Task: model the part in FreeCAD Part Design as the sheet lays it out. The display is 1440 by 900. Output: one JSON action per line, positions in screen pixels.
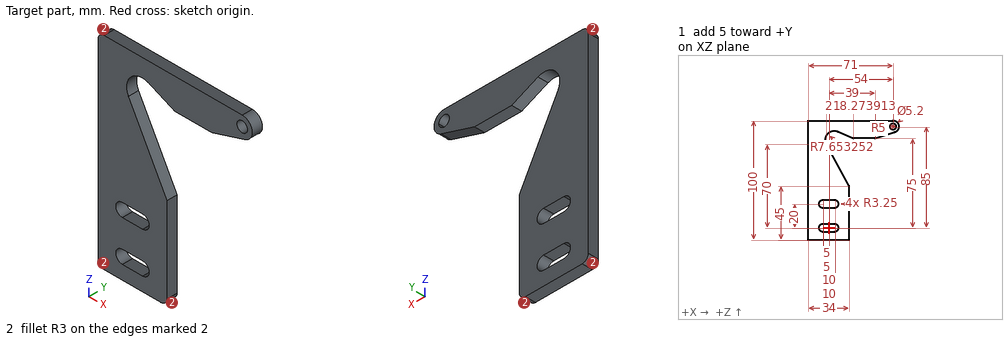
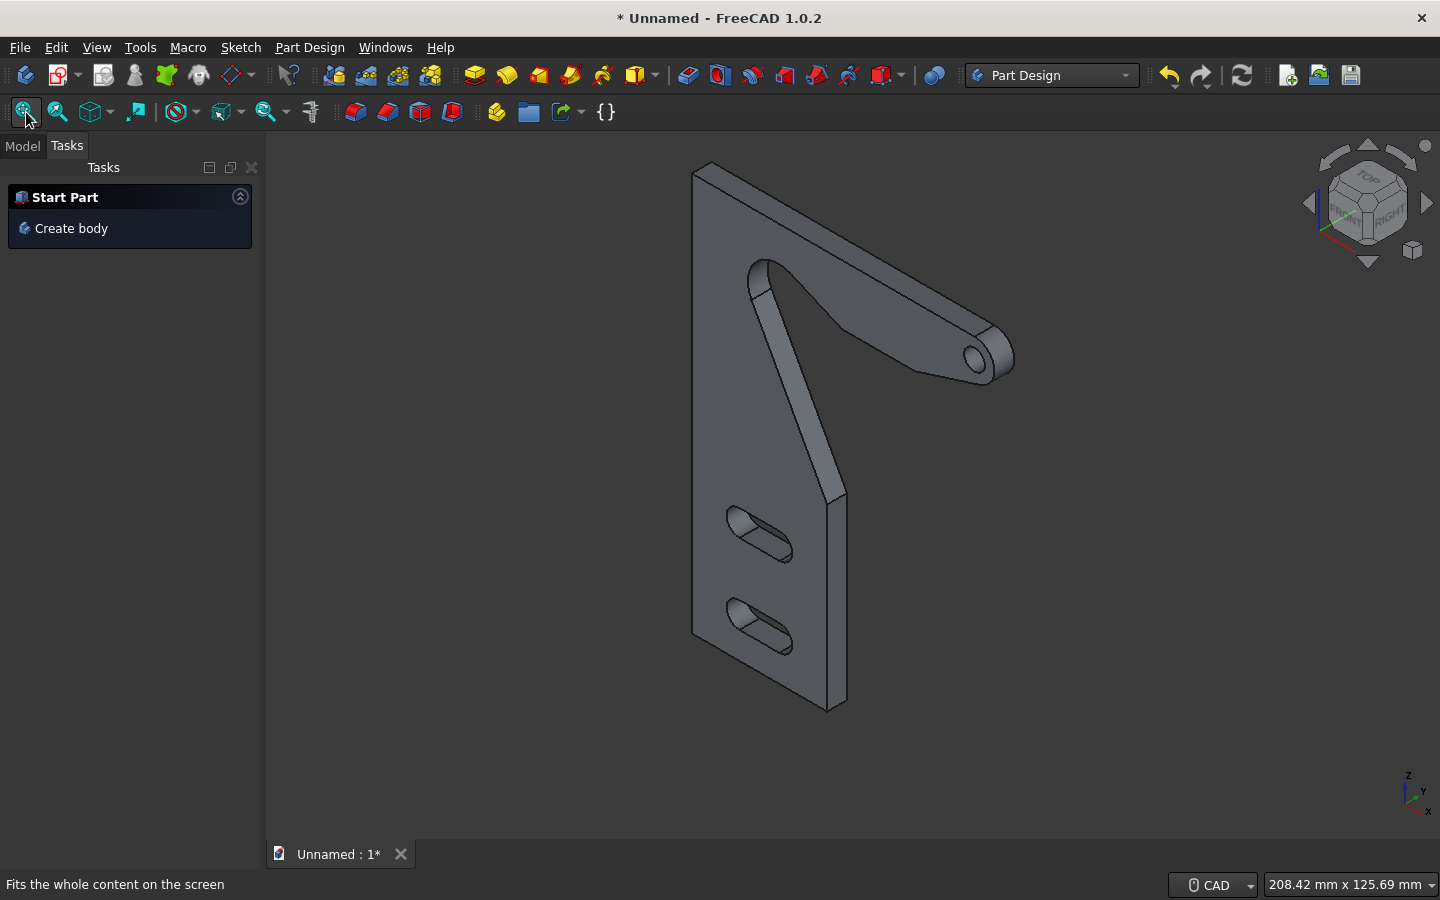
{"action": "key", "text": "2"}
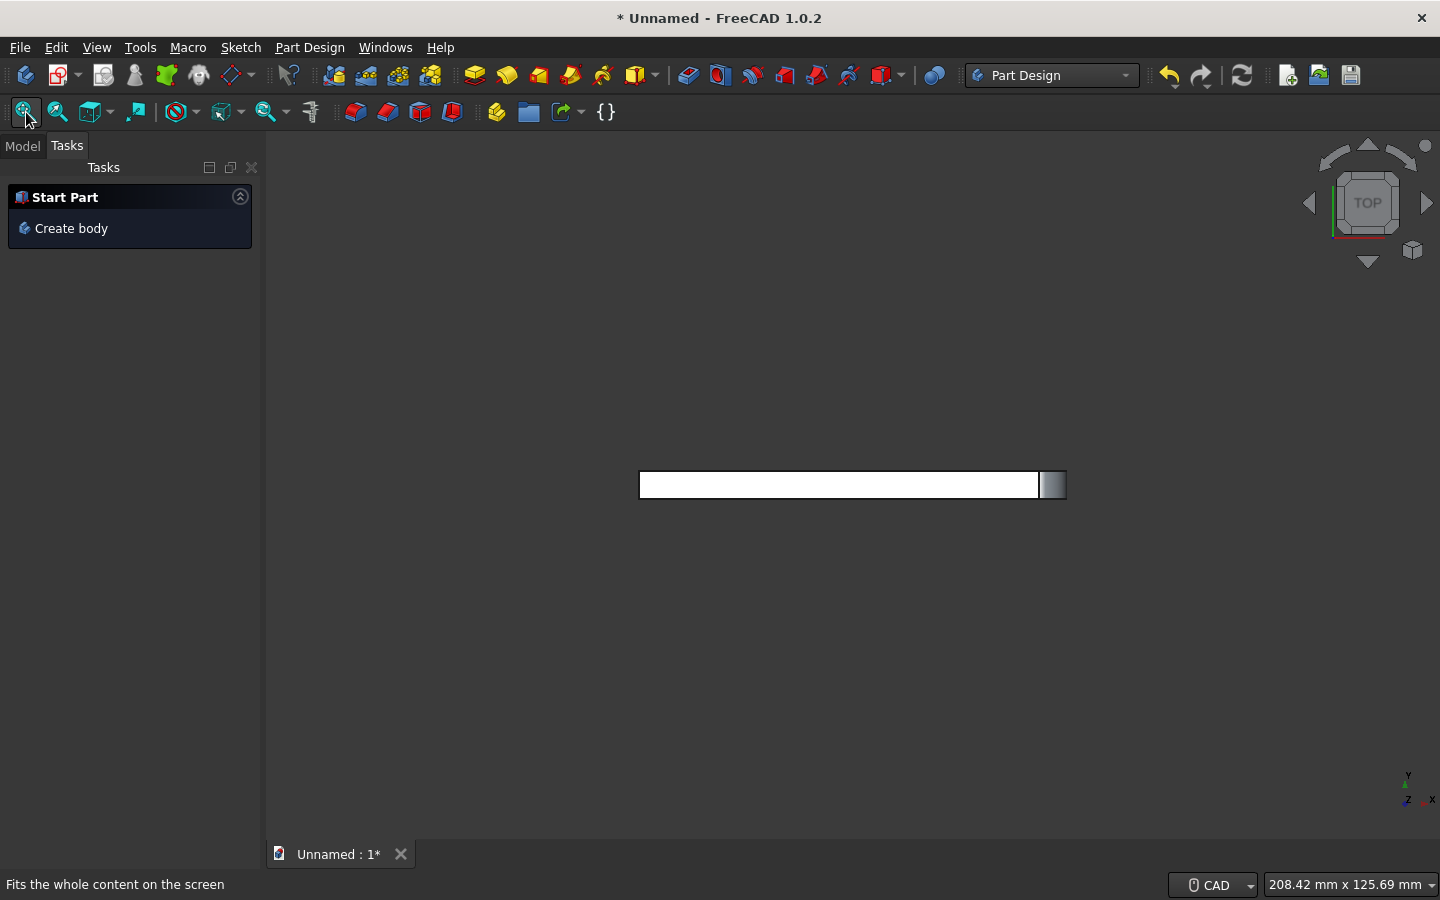
{"action": "left_click", "coordinate": [26, 112]}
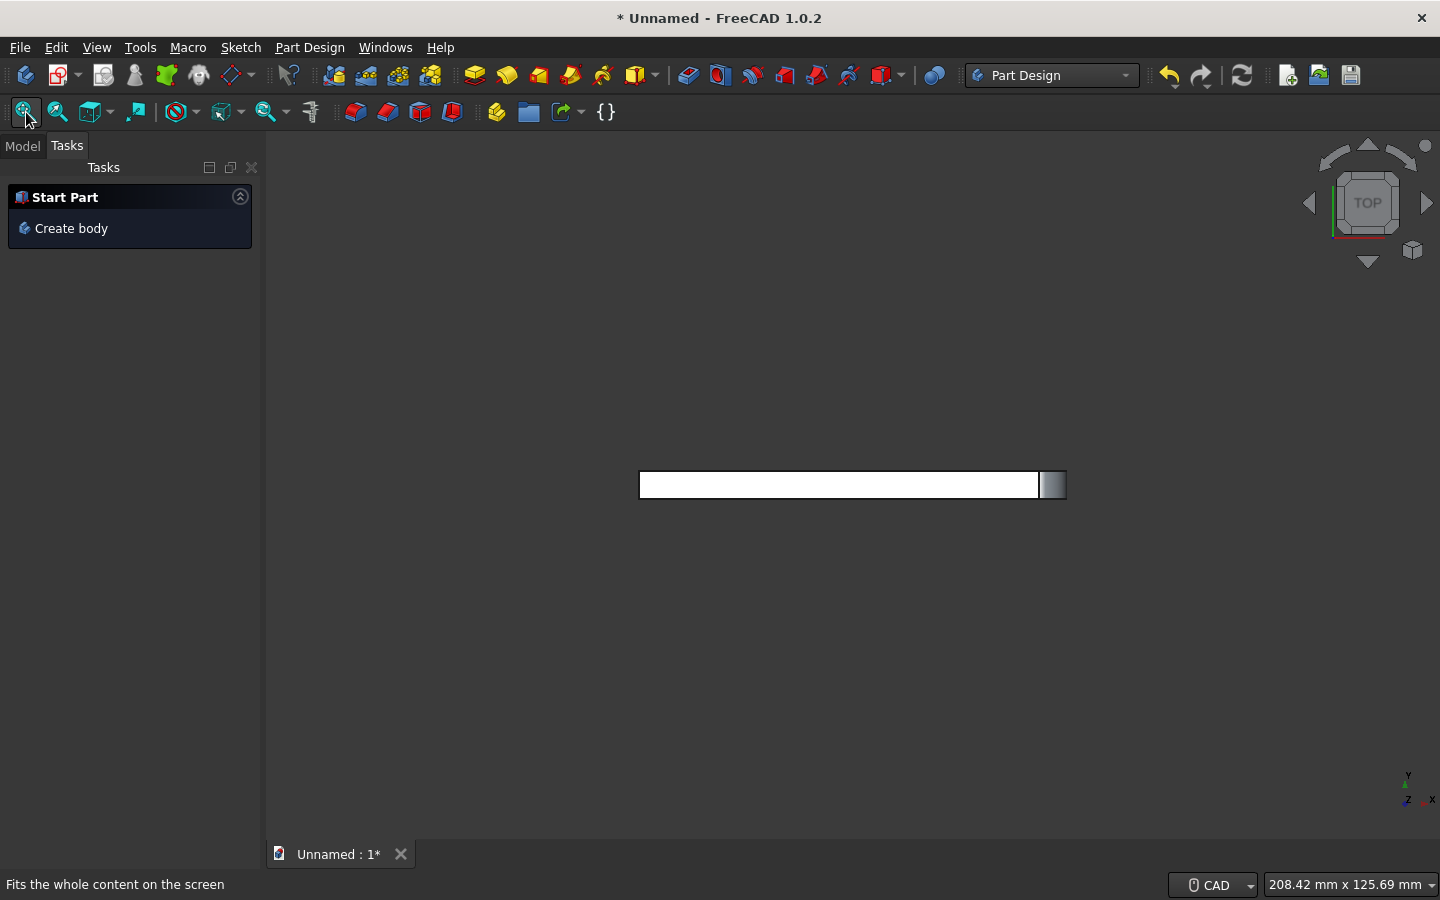
{"action": "left_click", "coordinate": [639, 484]}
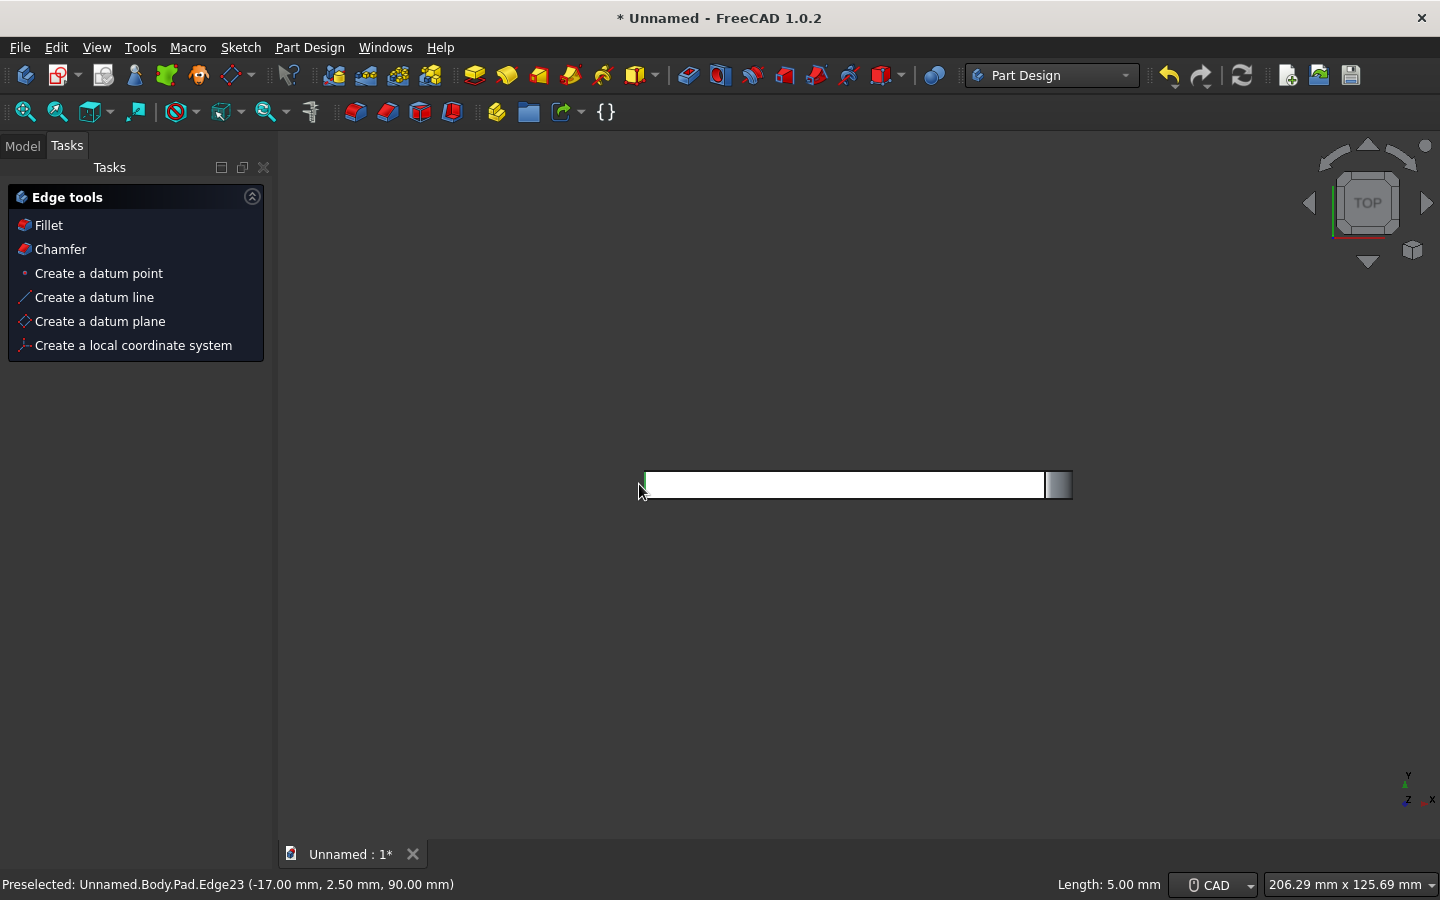
{"action": "key", "text": "1"}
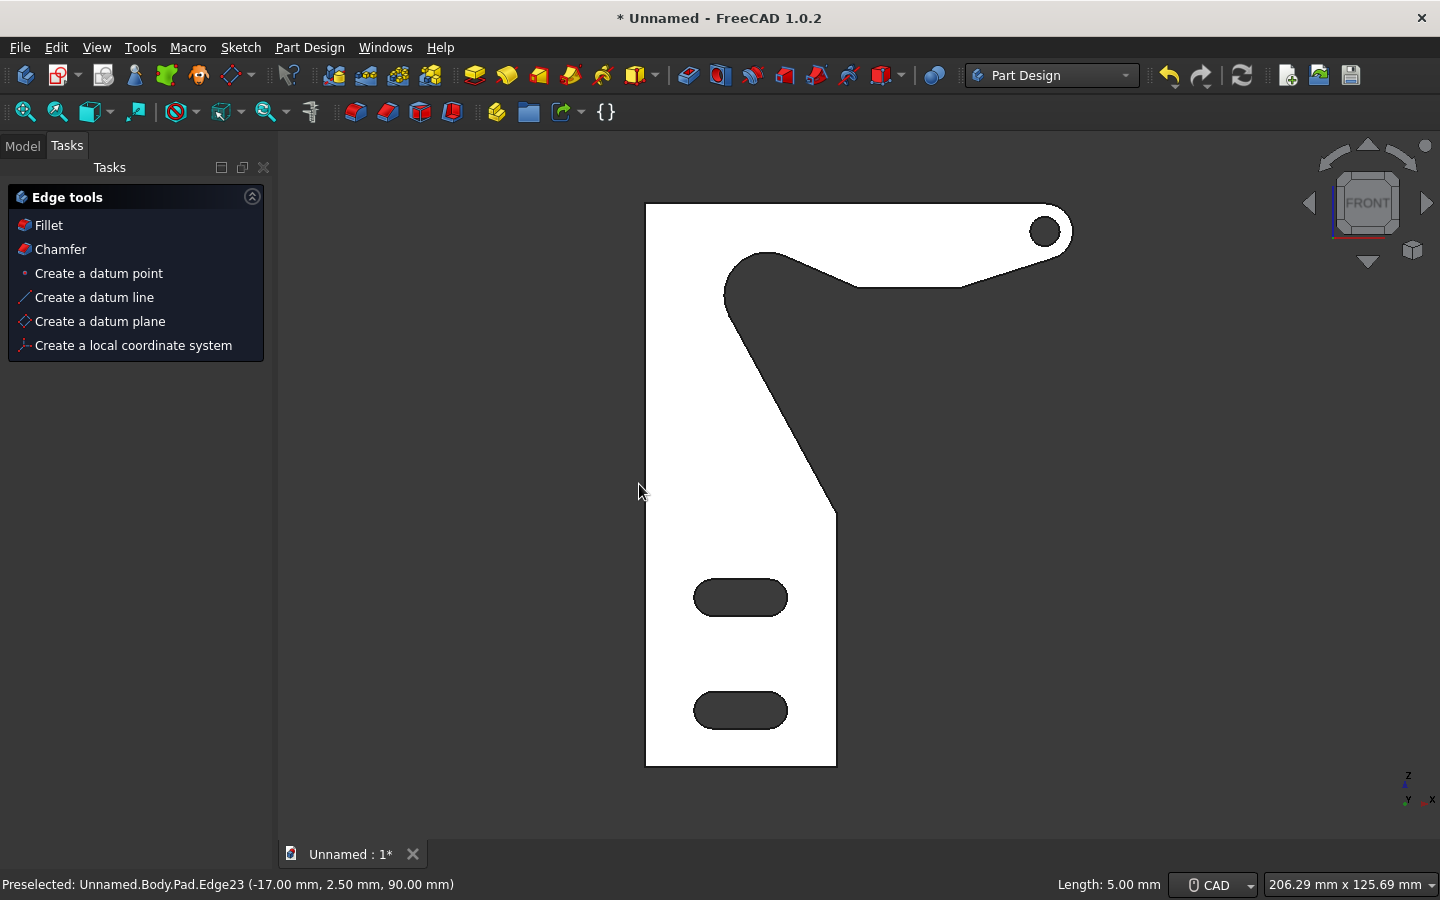
{"action": "key", "text": "3"}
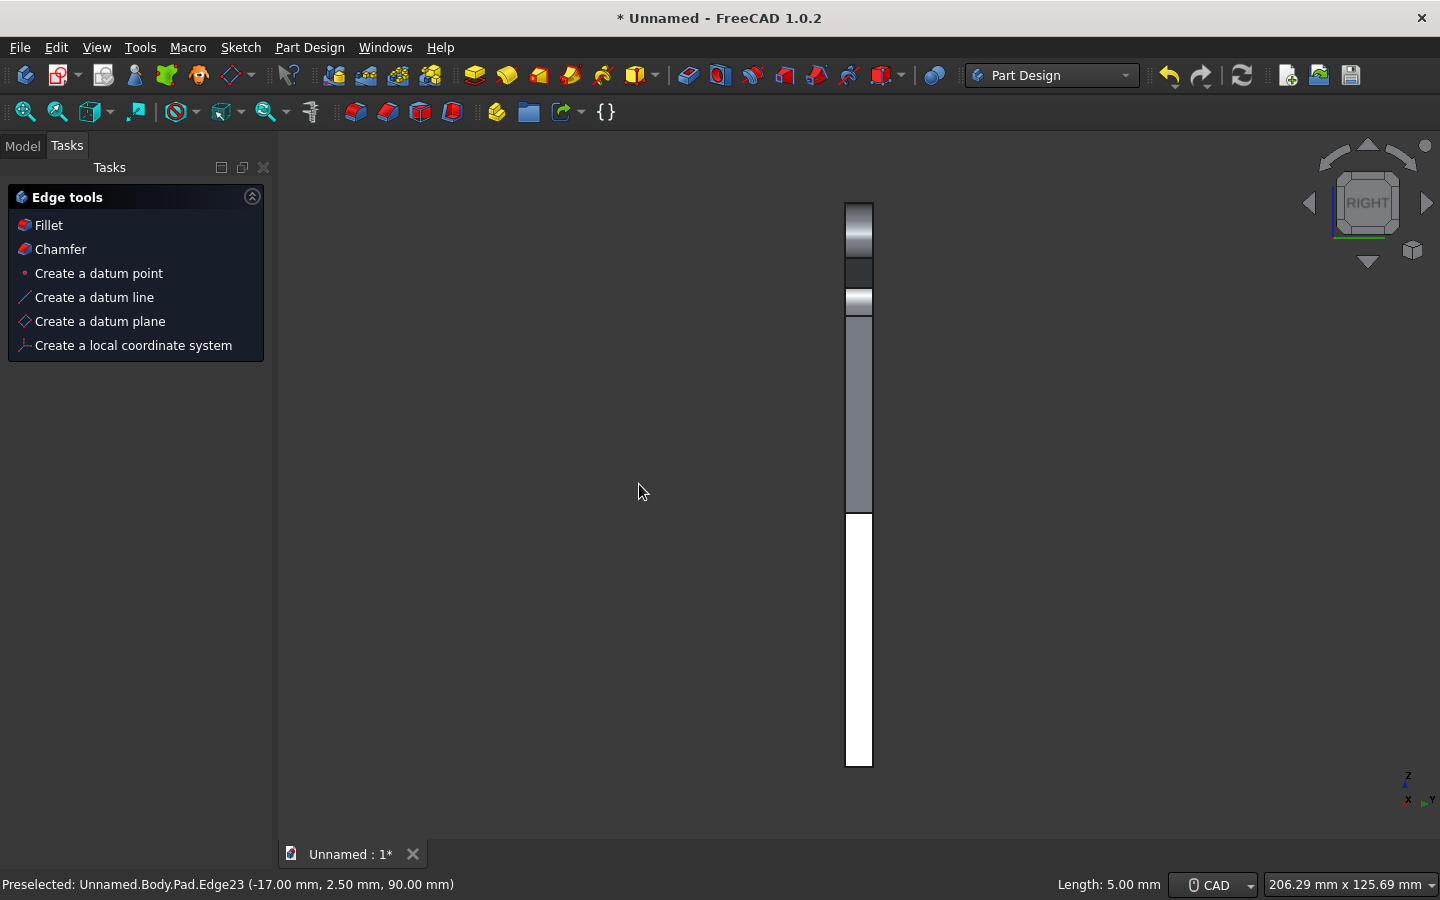
{"action": "left_click", "coordinate": [859, 766], "text": "ctrl"}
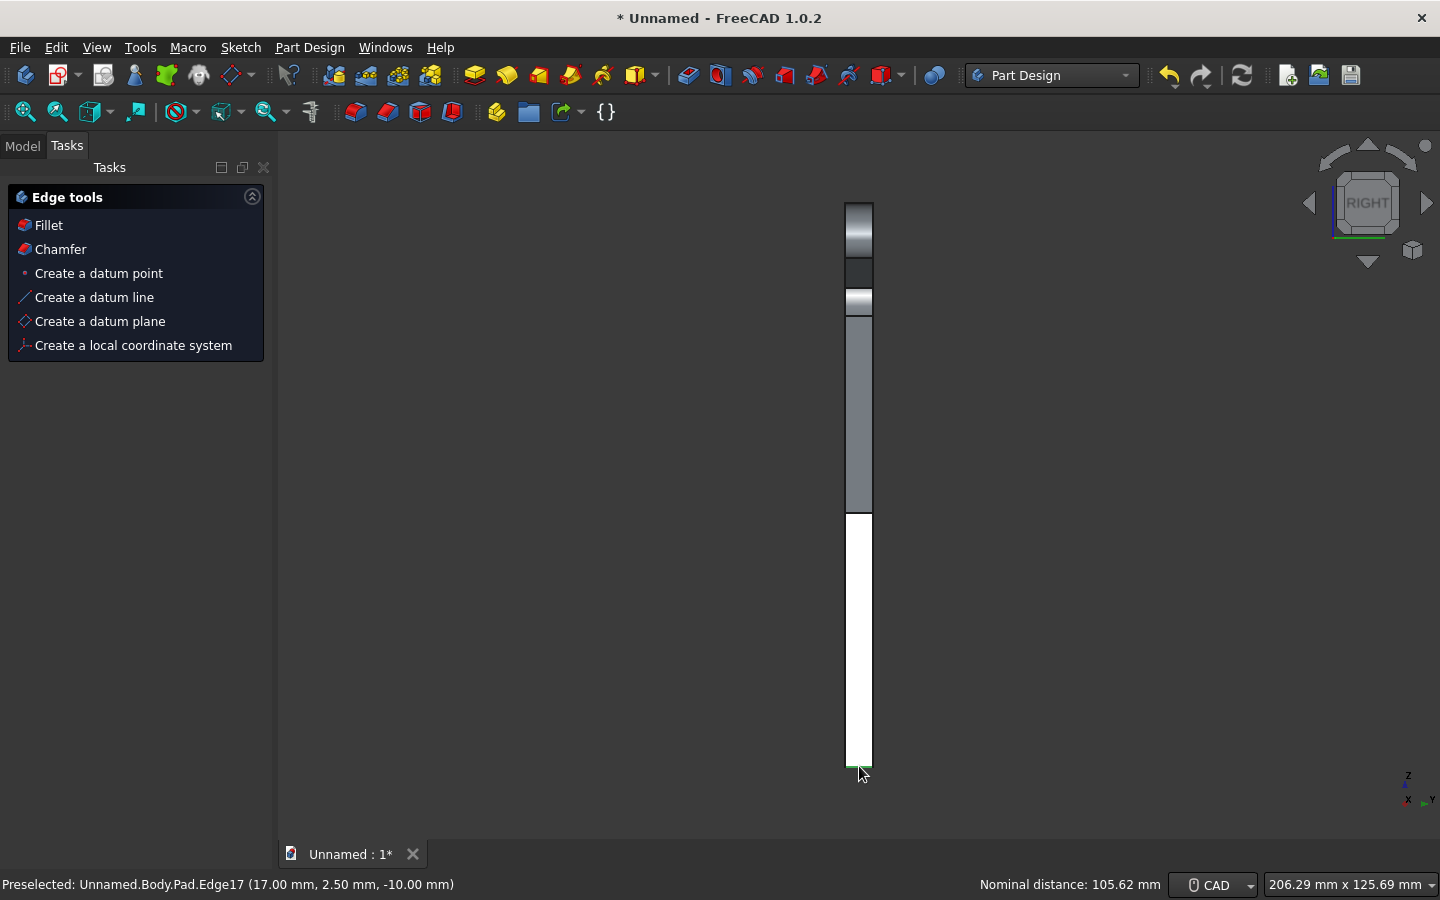
{"action": "key", "text": "5"}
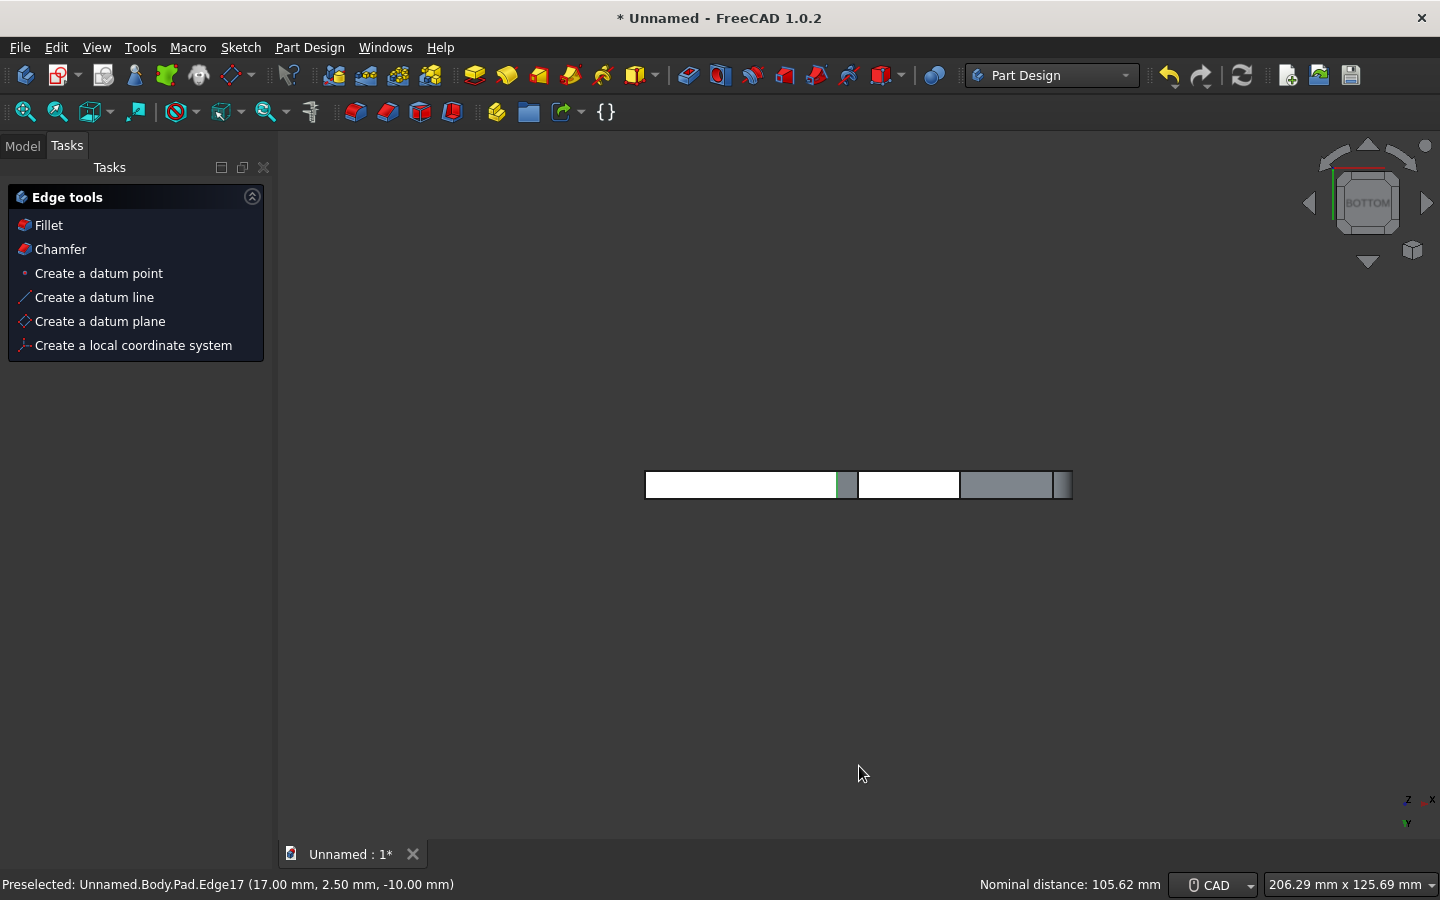
{"action": "left_click", "coordinate": [26, 112]}